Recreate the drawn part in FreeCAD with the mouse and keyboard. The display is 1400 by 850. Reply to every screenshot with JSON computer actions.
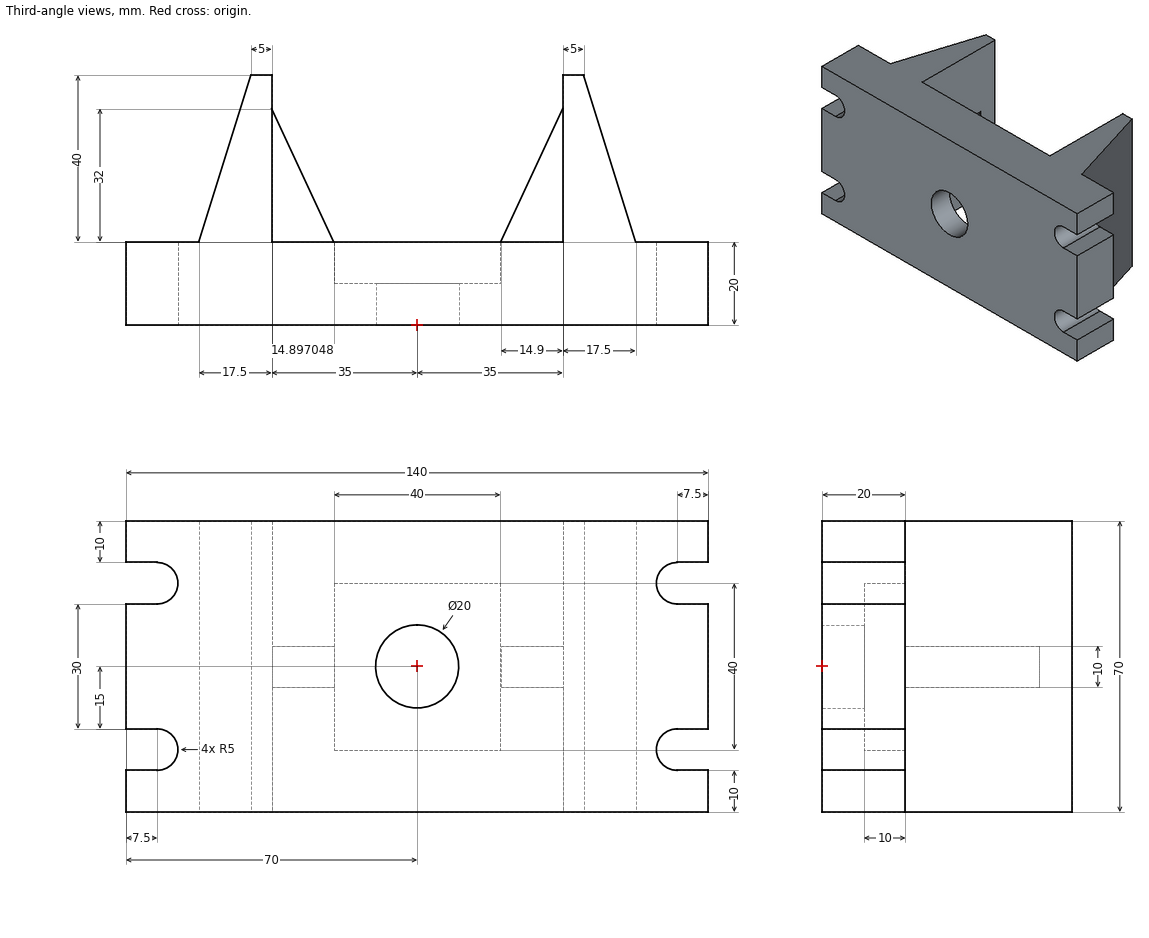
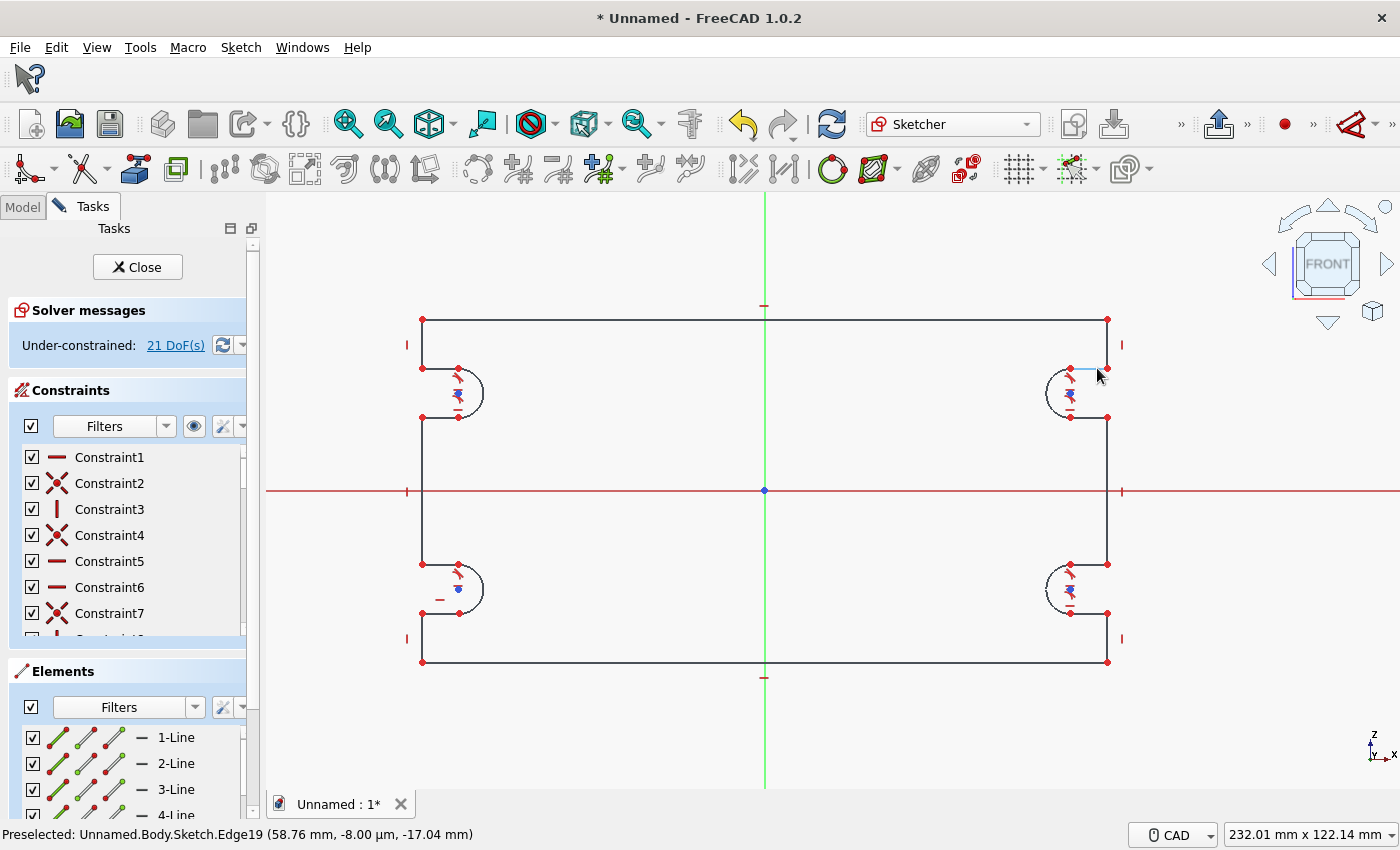
{"action": "scroll", "coordinate": [433, 614], "scroll_direction": "up", "scroll_amount": 2}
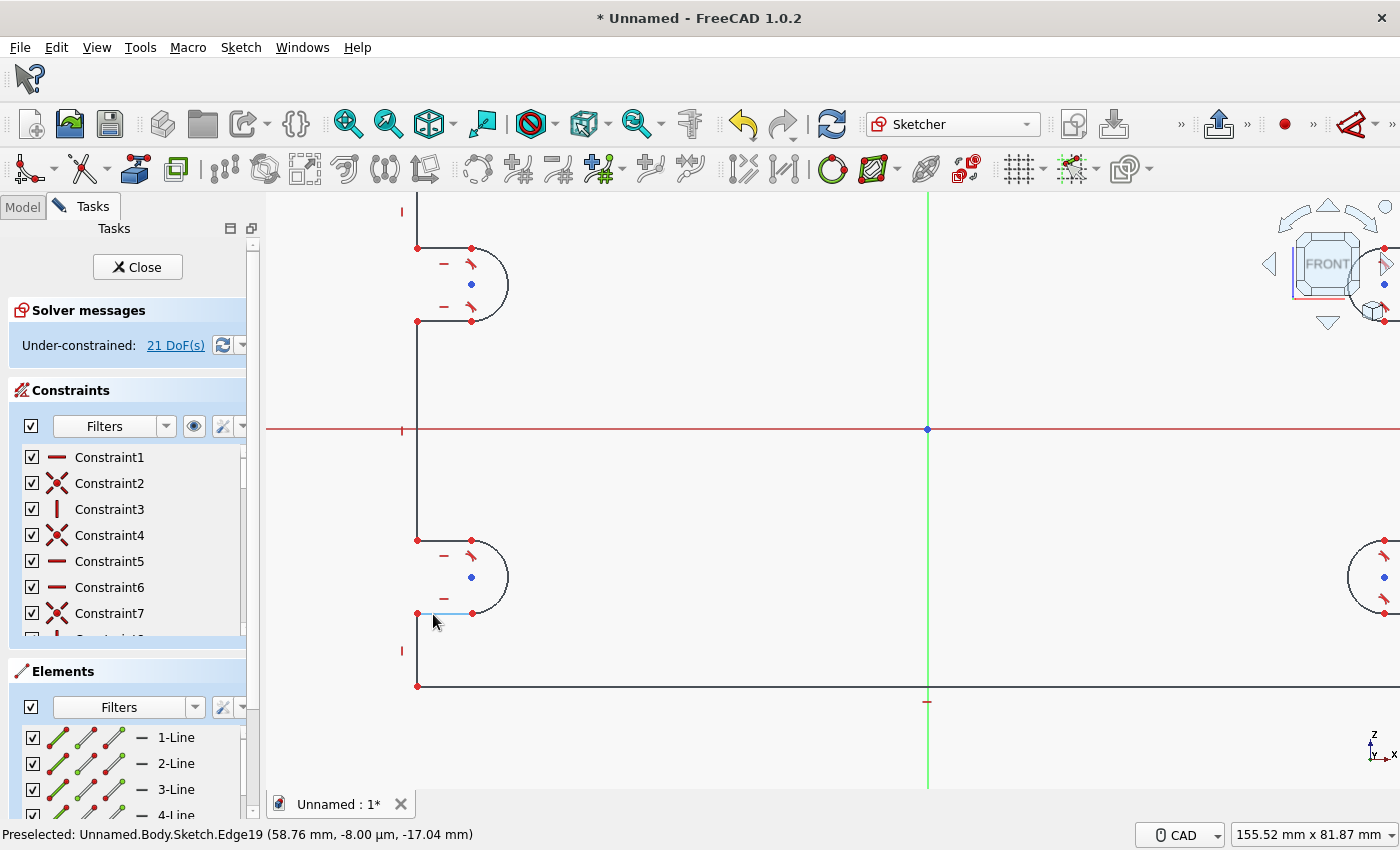
{"action": "left_click", "coordinate": [434, 614]}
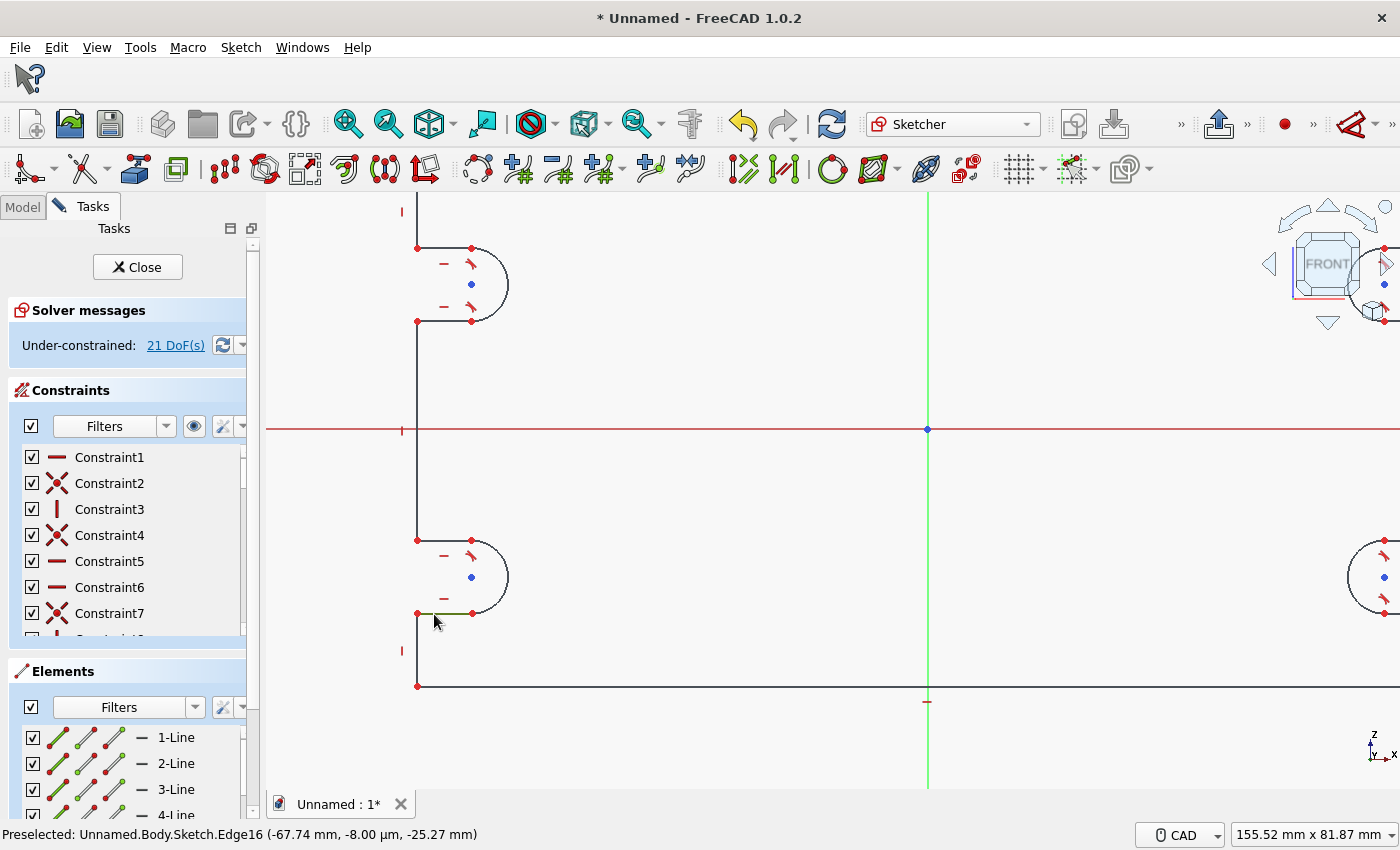
{"action": "left_click", "coordinate": [501, 598]}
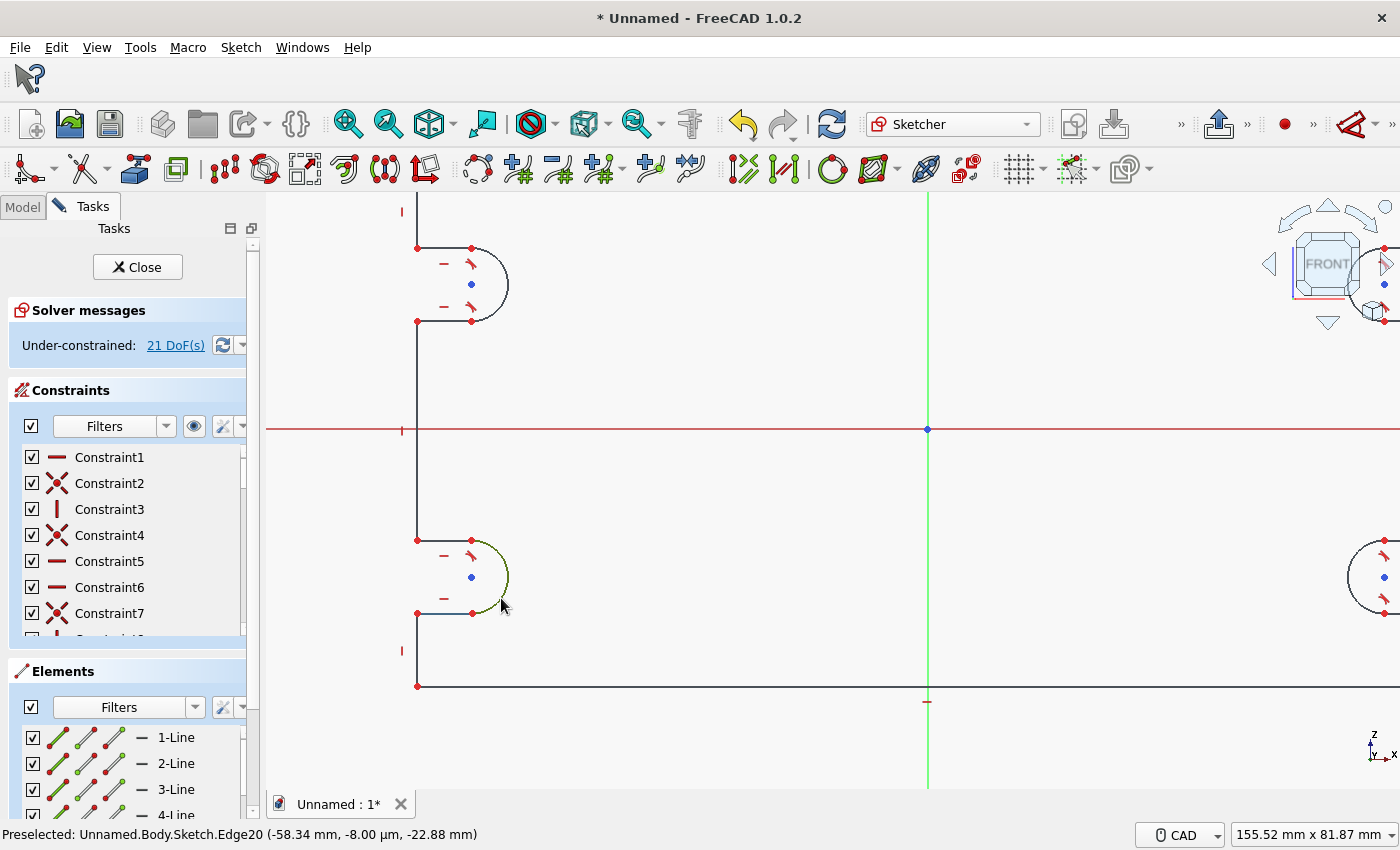
{"action": "key", "text": "t"}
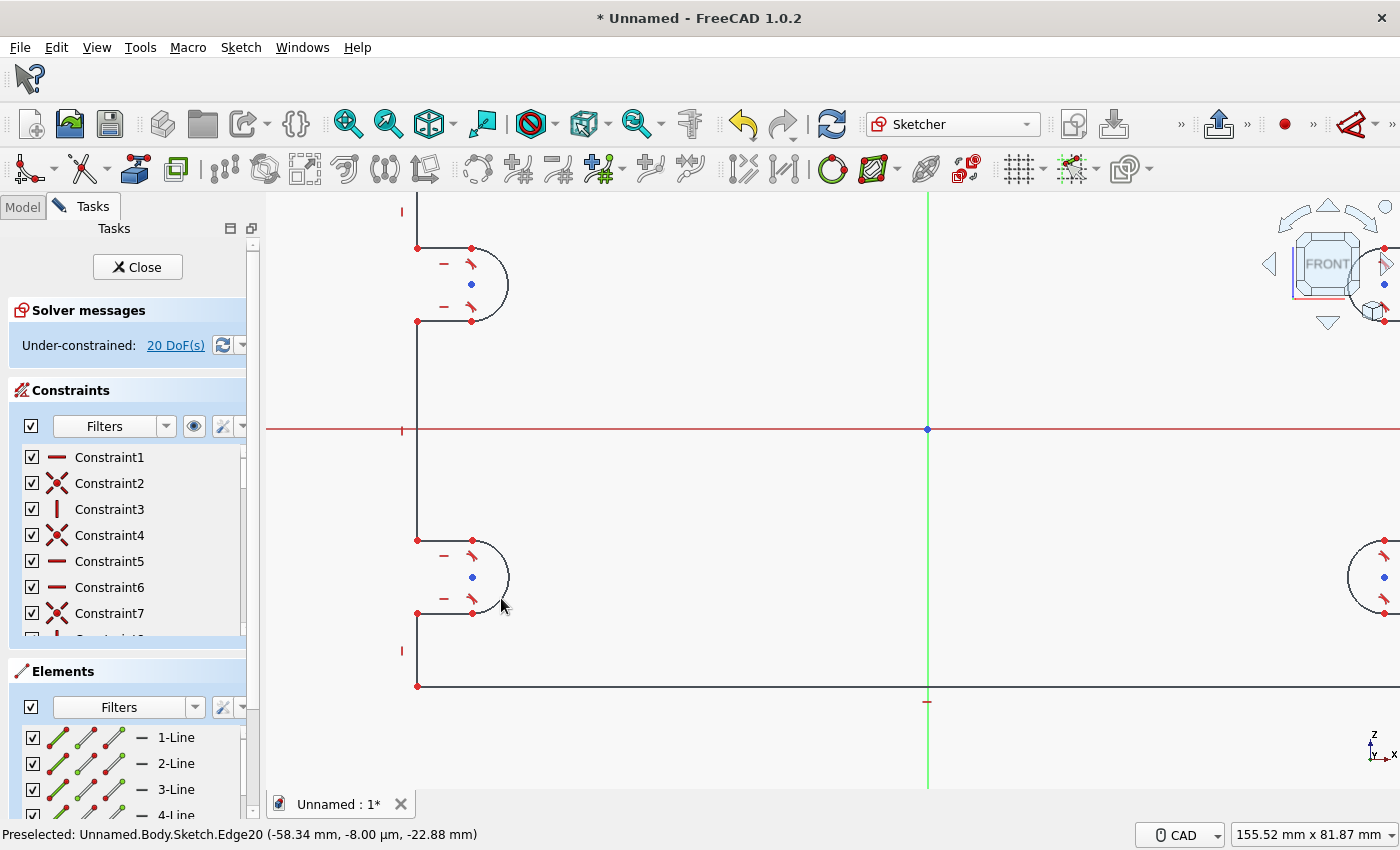
{"action": "left_click", "coordinate": [501, 306]}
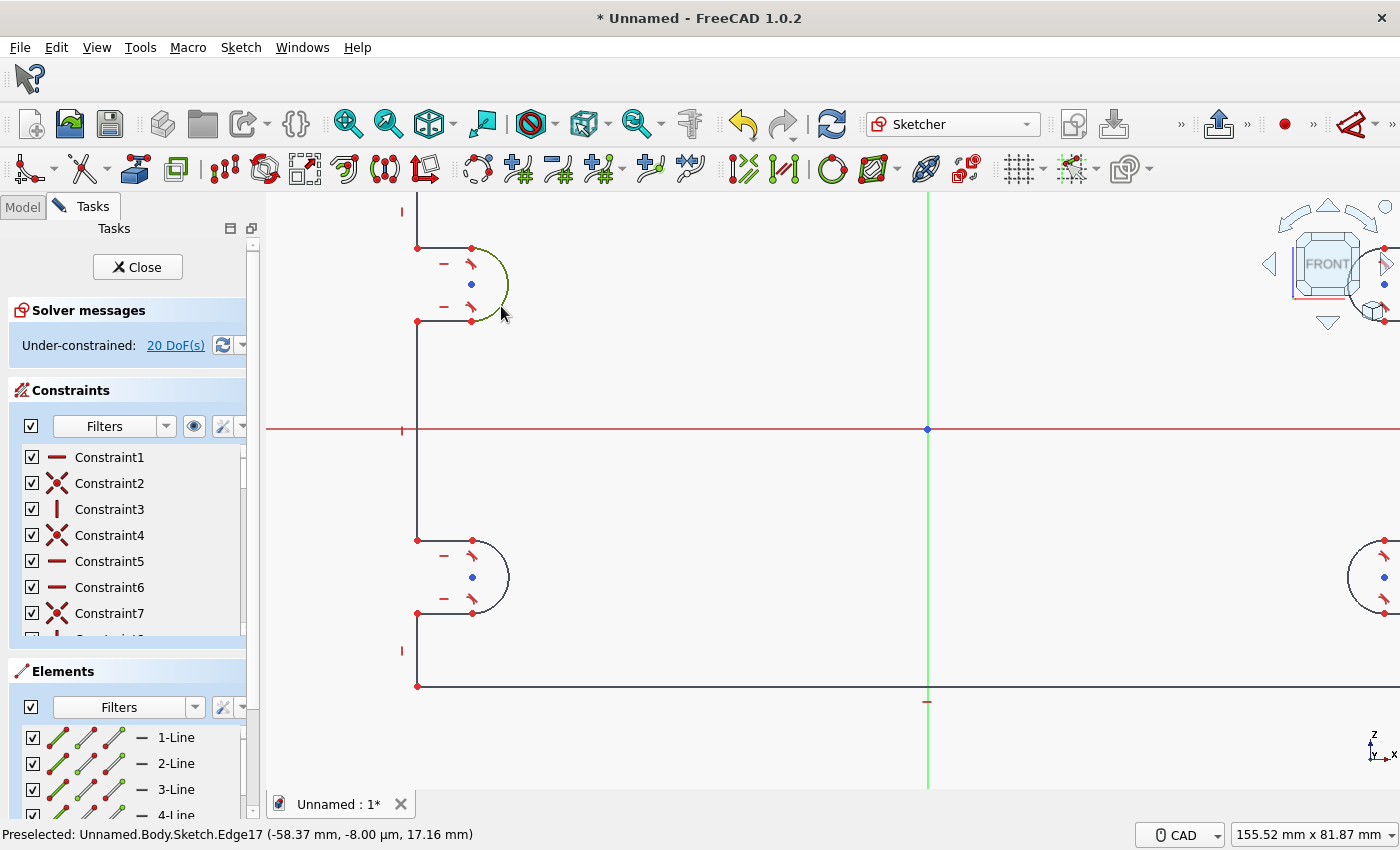
{"action": "scroll", "coordinate": [432, 615], "scroll_direction": "down", "scroll_amount": 2}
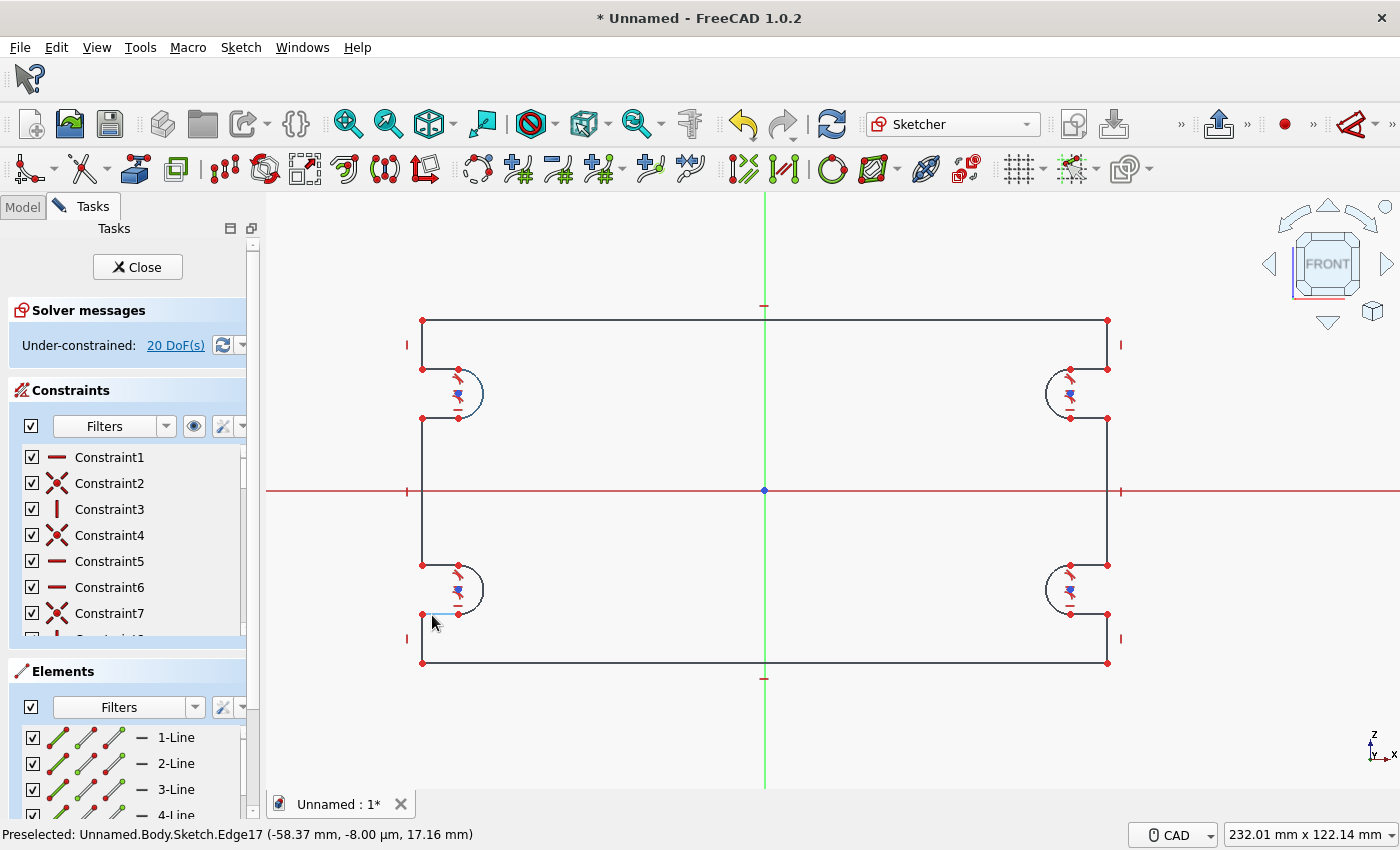
{"action": "left_click", "coordinate": [1051, 379]}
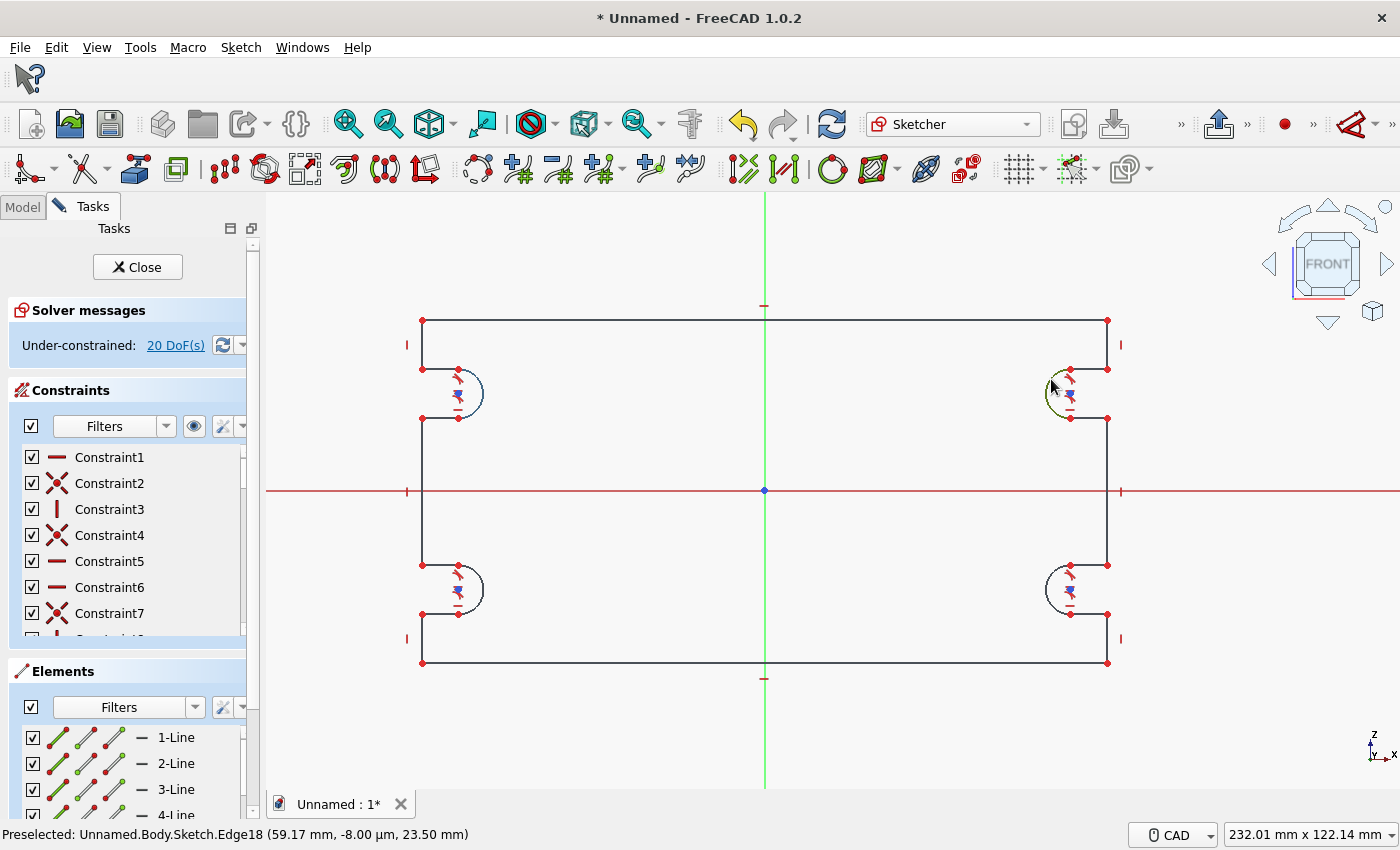
{"action": "left_click", "coordinate": [1051, 575]}